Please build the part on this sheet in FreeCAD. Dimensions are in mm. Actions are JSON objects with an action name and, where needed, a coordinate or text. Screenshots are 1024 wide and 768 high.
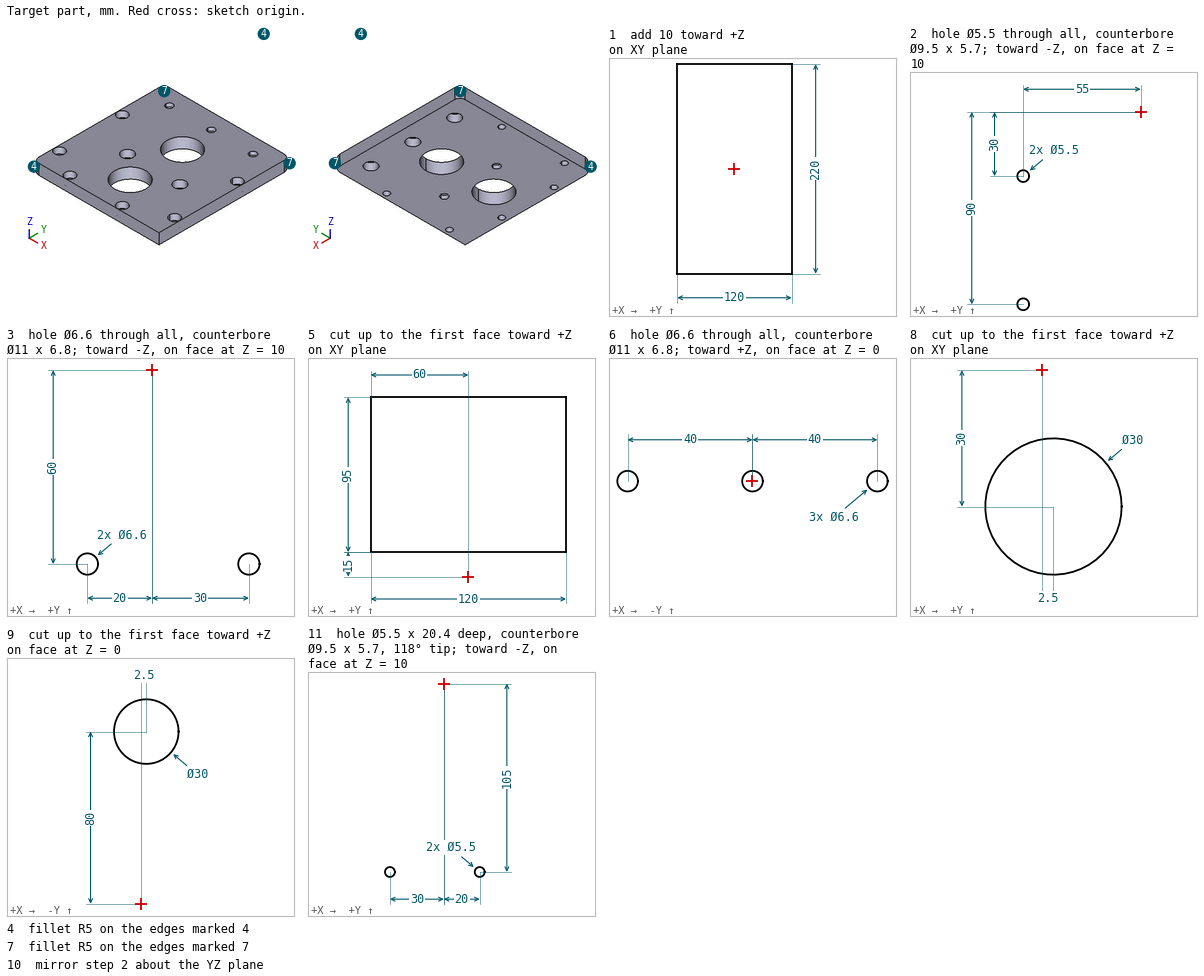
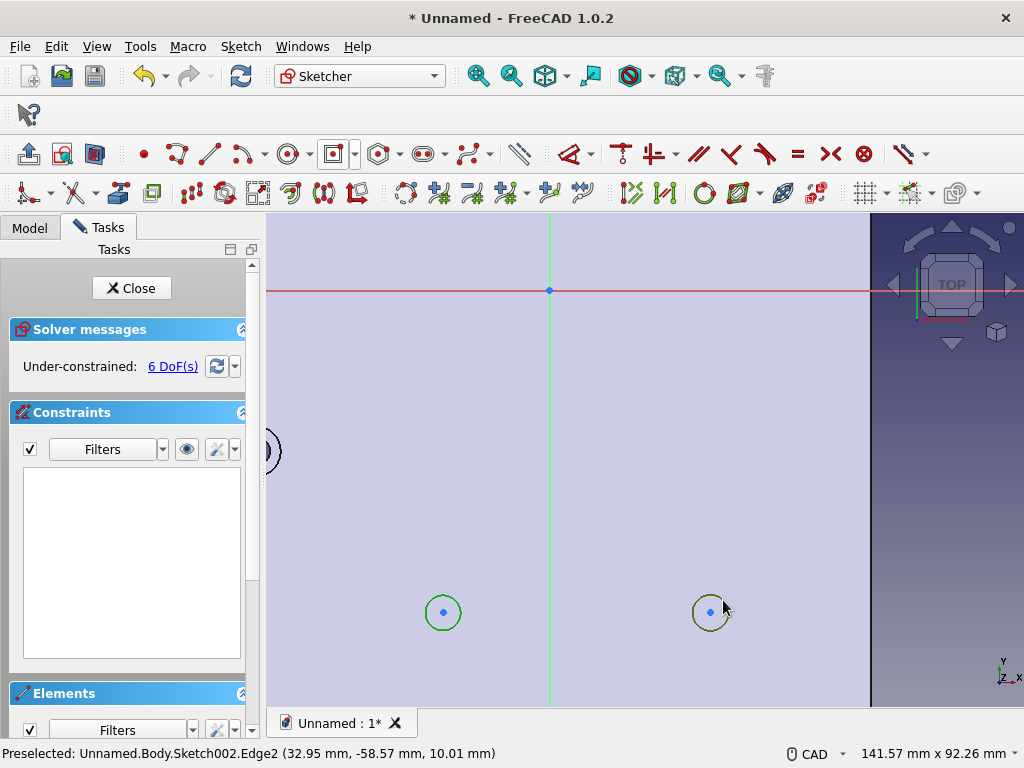
{"action": "left_click", "coordinate": [798, 154]}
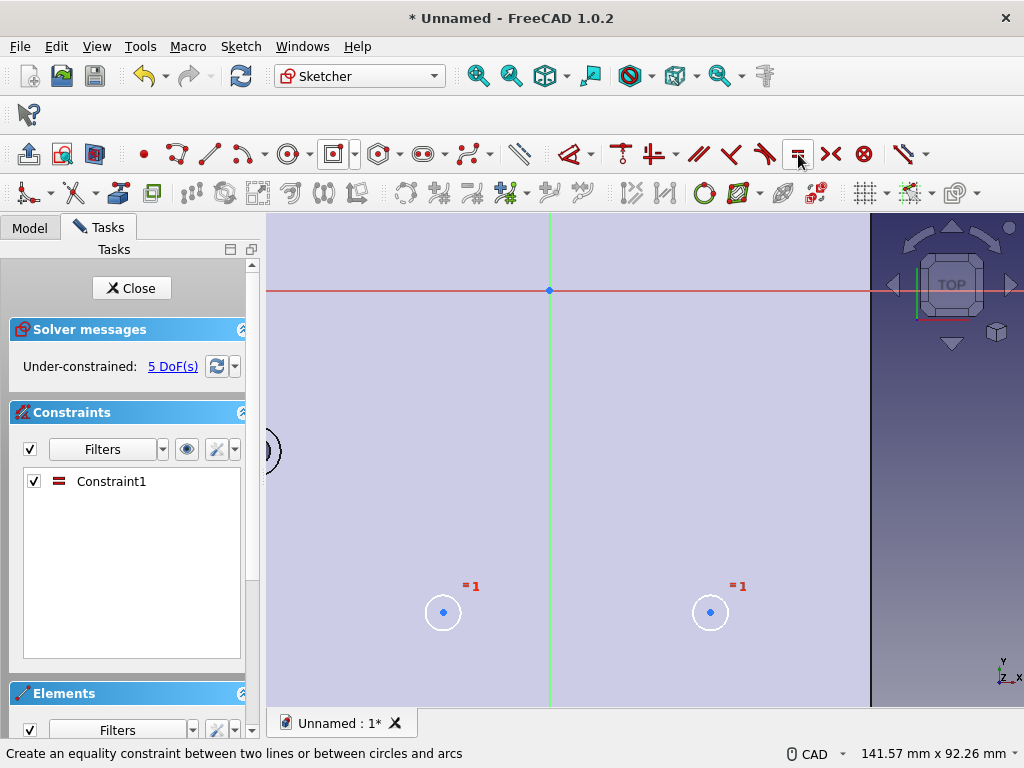
{"action": "left_click", "coordinate": [443, 613]}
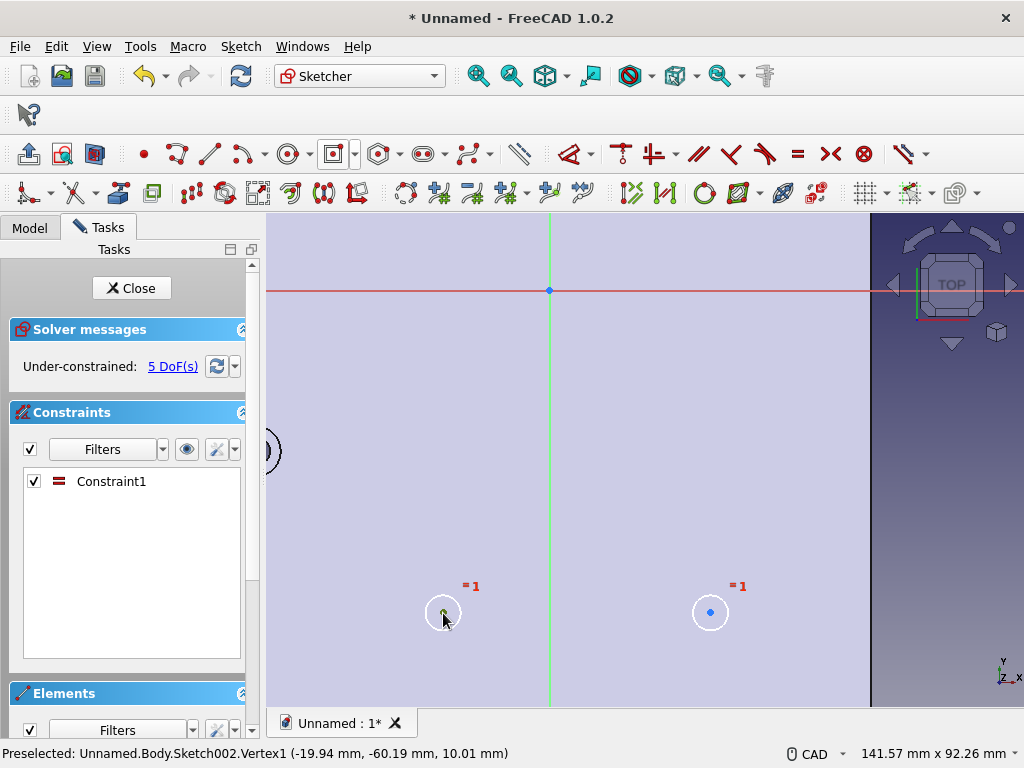
{"action": "left_click", "coordinate": [711, 613]}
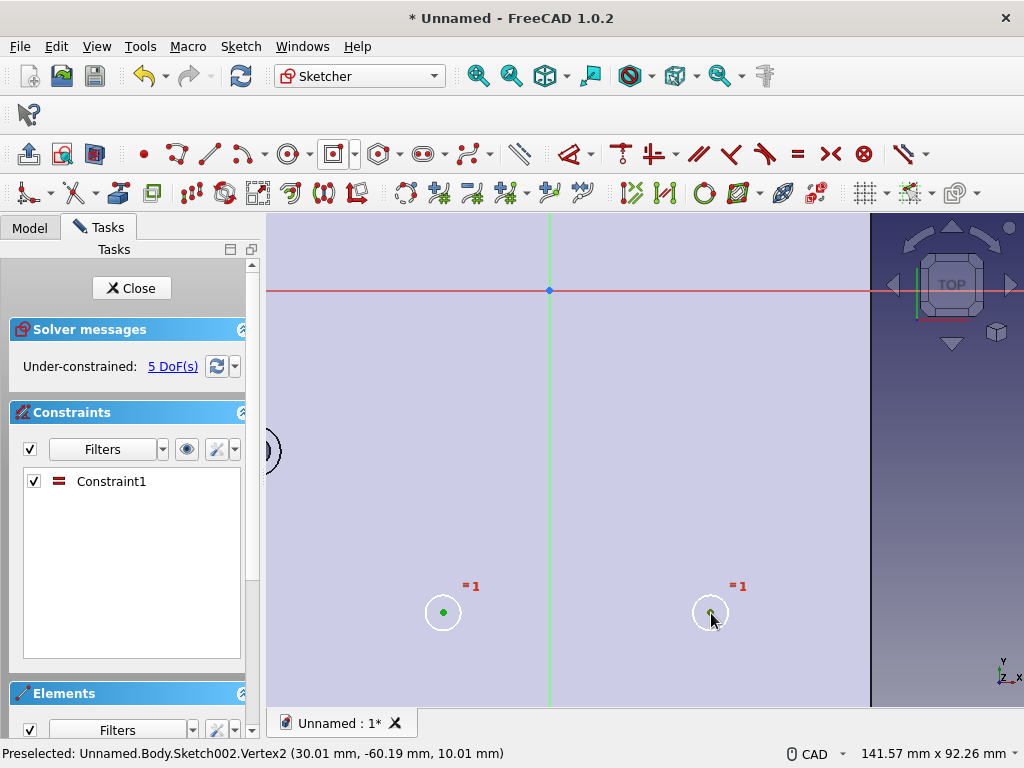
{"action": "left_click", "coordinate": [676, 154]}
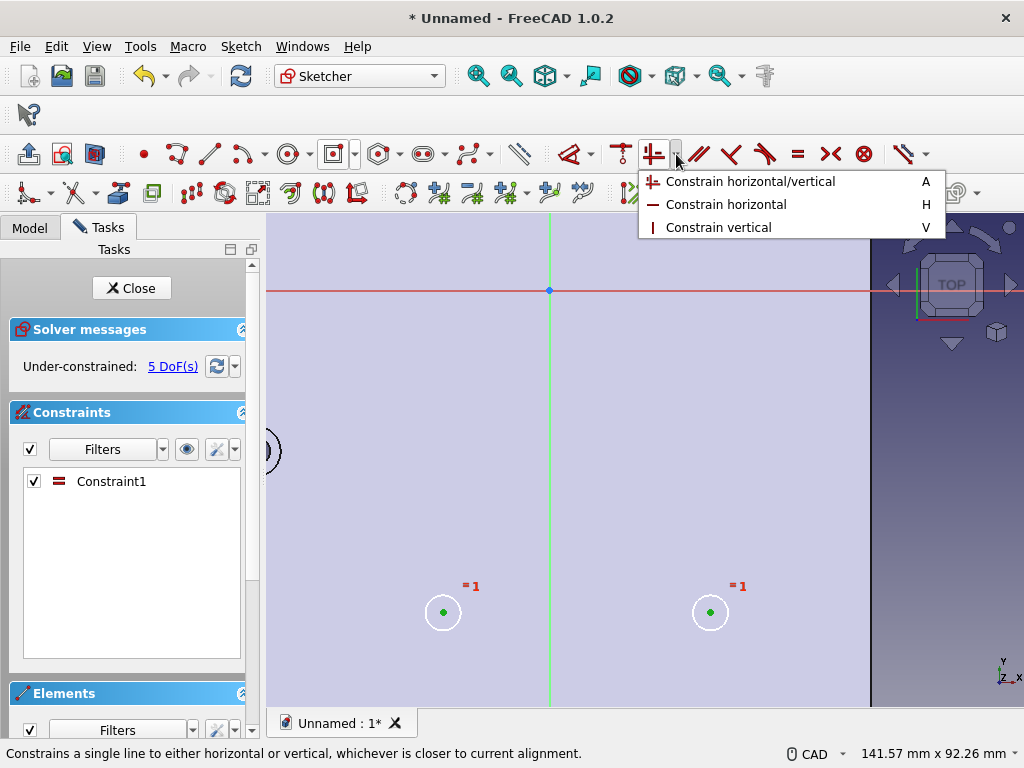
{"action": "left_click", "coordinate": [792, 204]}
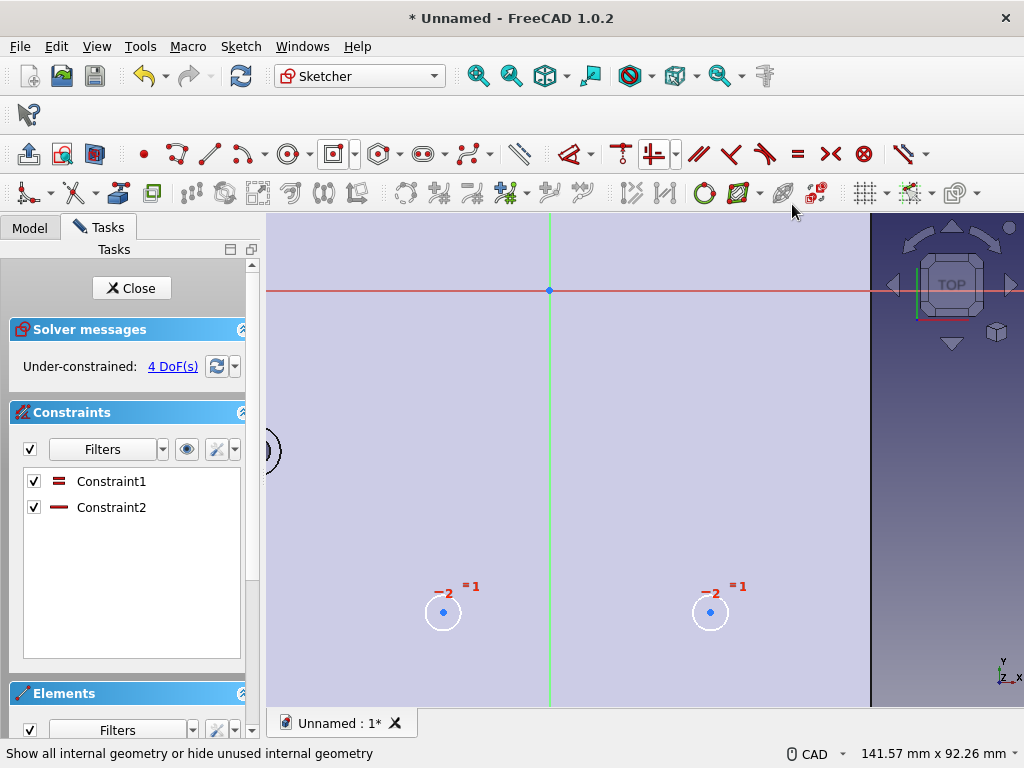
{"action": "left_click", "coordinate": [568, 154]}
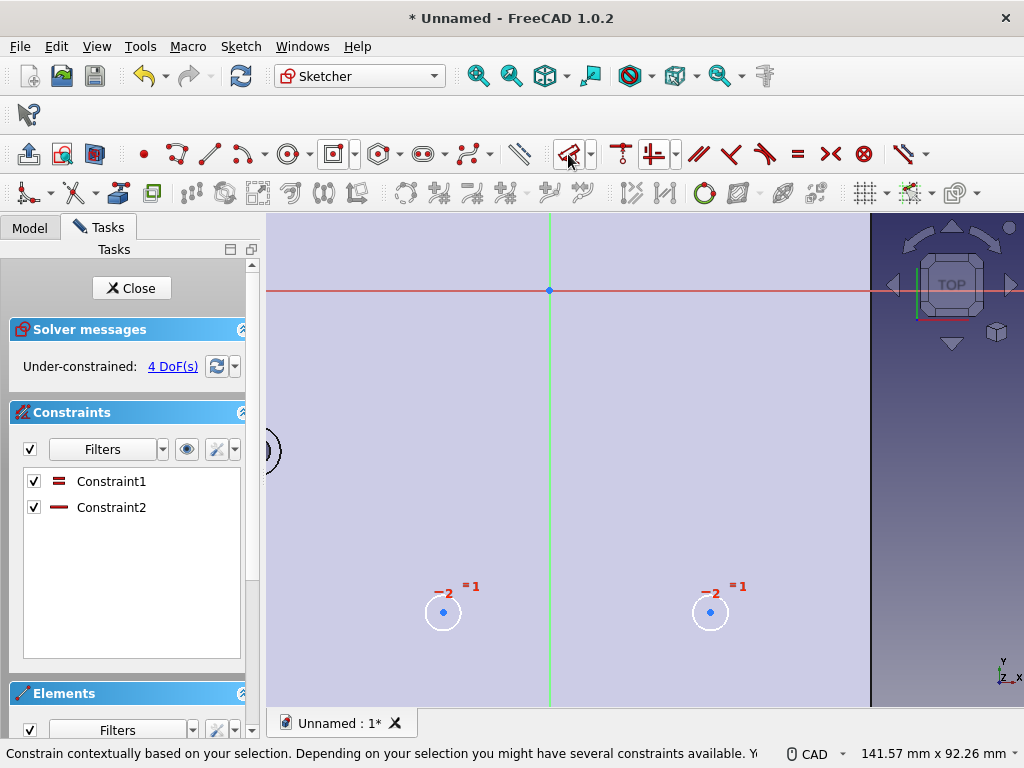
{"action": "left_click", "coordinate": [455, 600]}
{"action": "left_click", "coordinate": [477, 576]}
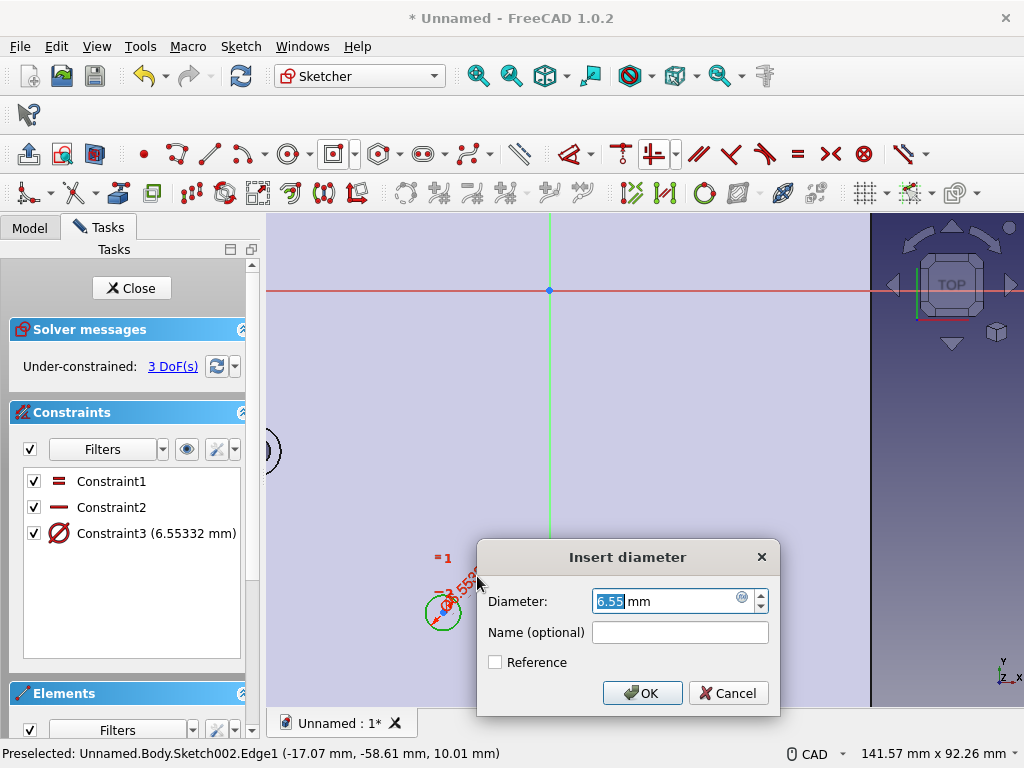
{"action": "type", "text": "6.6"}
{"action": "key", "text": "Return"}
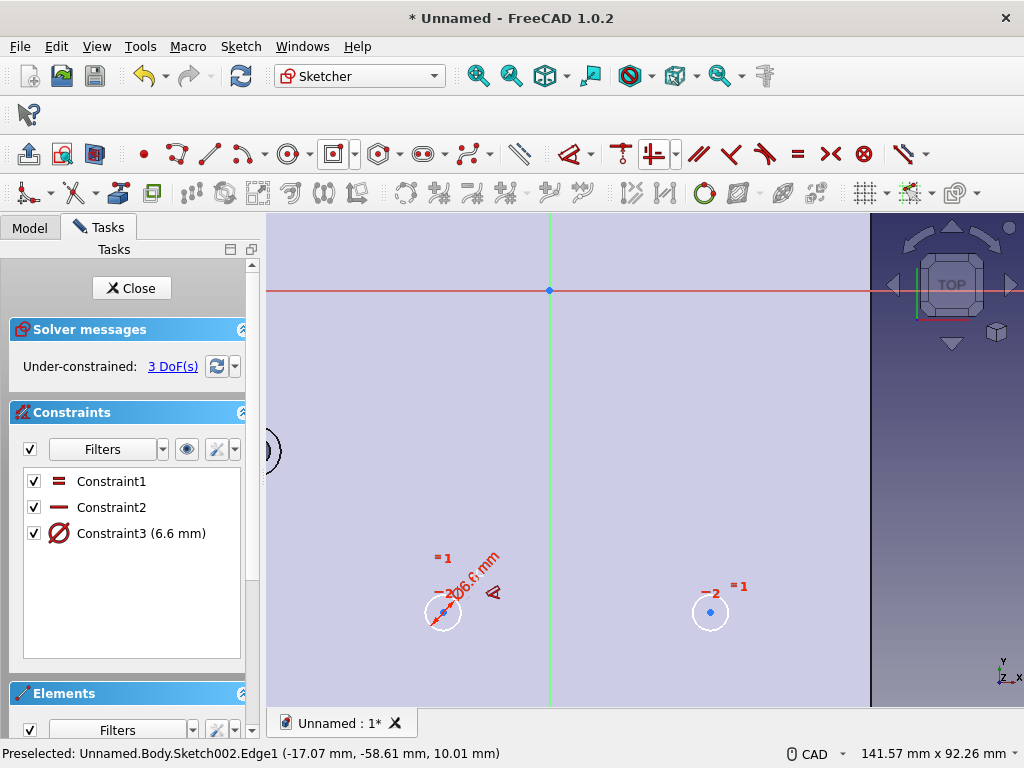
{"action": "left_click", "coordinate": [443, 613]}
{"action": "left_click", "coordinate": [496, 257]}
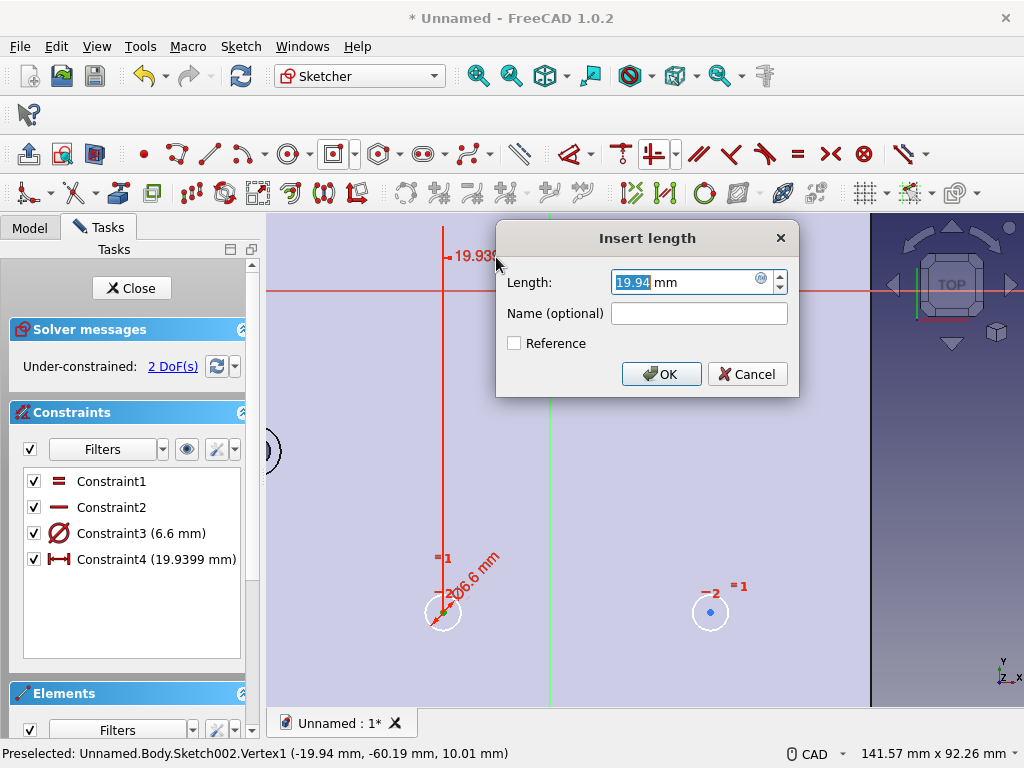
{"action": "type", "text": "20"}
{"action": "key", "text": "Return"}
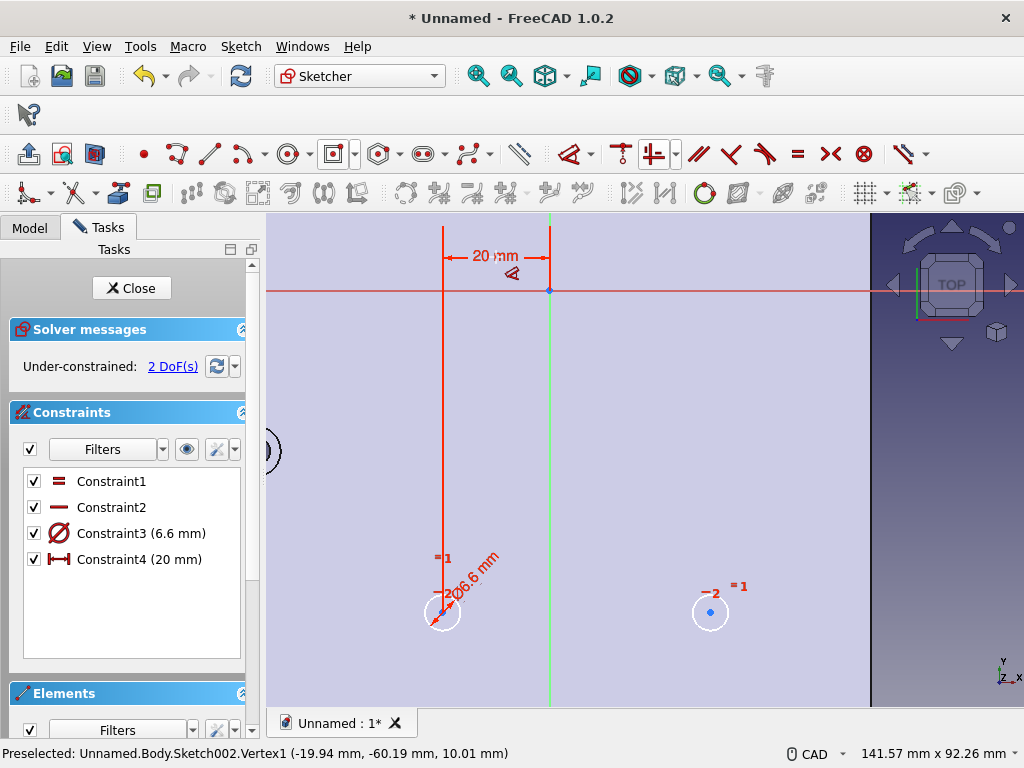
{"action": "left_click", "coordinate": [443, 613]}
{"action": "left_click", "coordinate": [409, 452]}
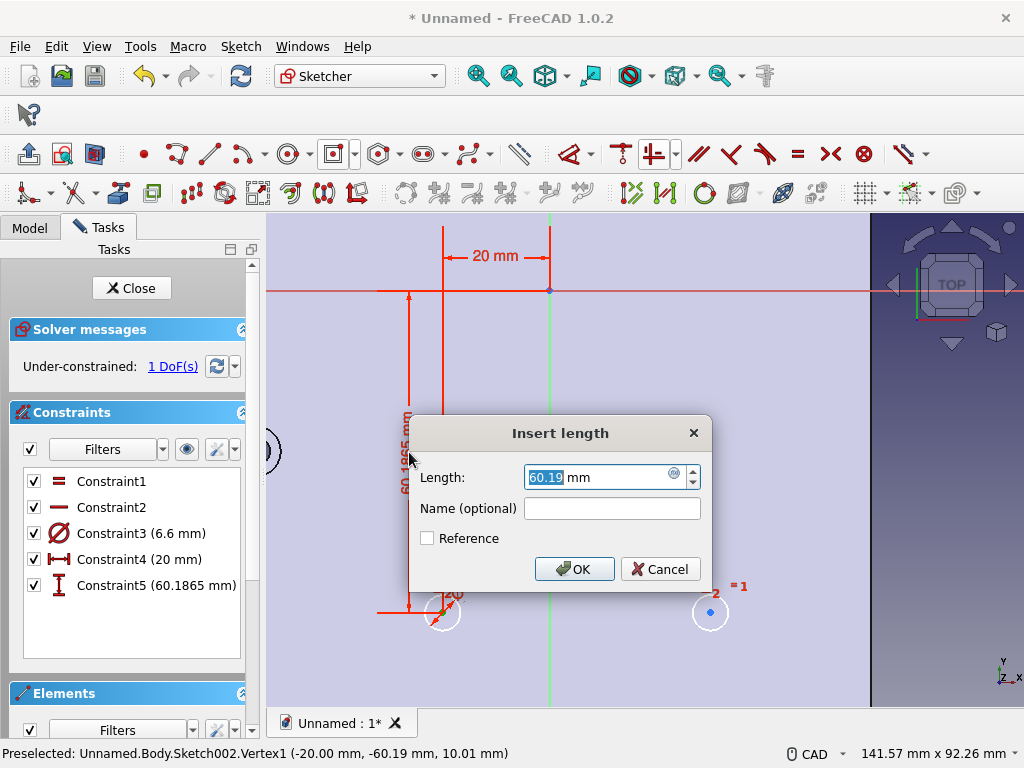
{"action": "type", "text": "60"}
{"action": "key", "text": "Return"}